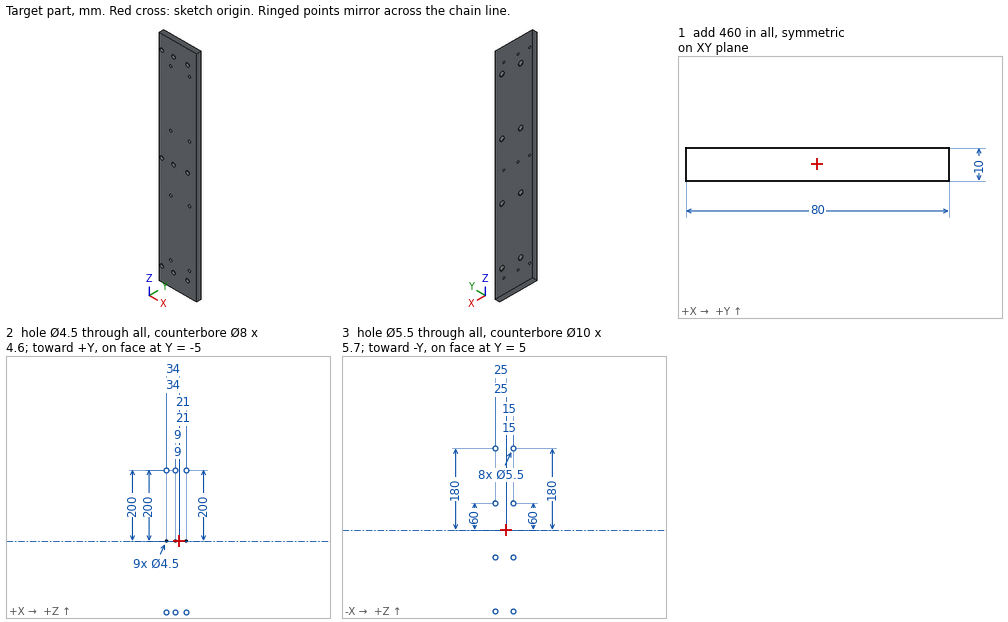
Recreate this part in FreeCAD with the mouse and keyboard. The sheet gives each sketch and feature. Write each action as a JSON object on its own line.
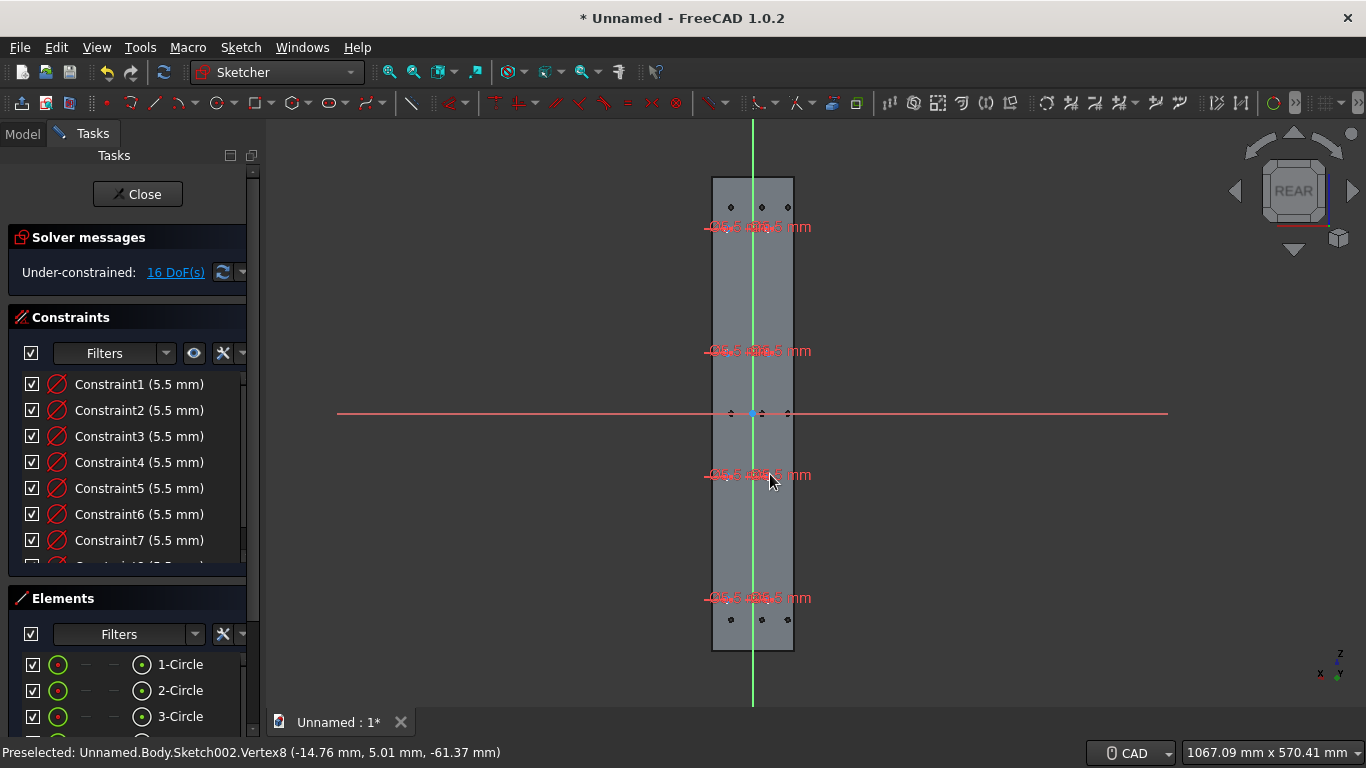
{"action": "left_click", "coordinate": [727, 353]}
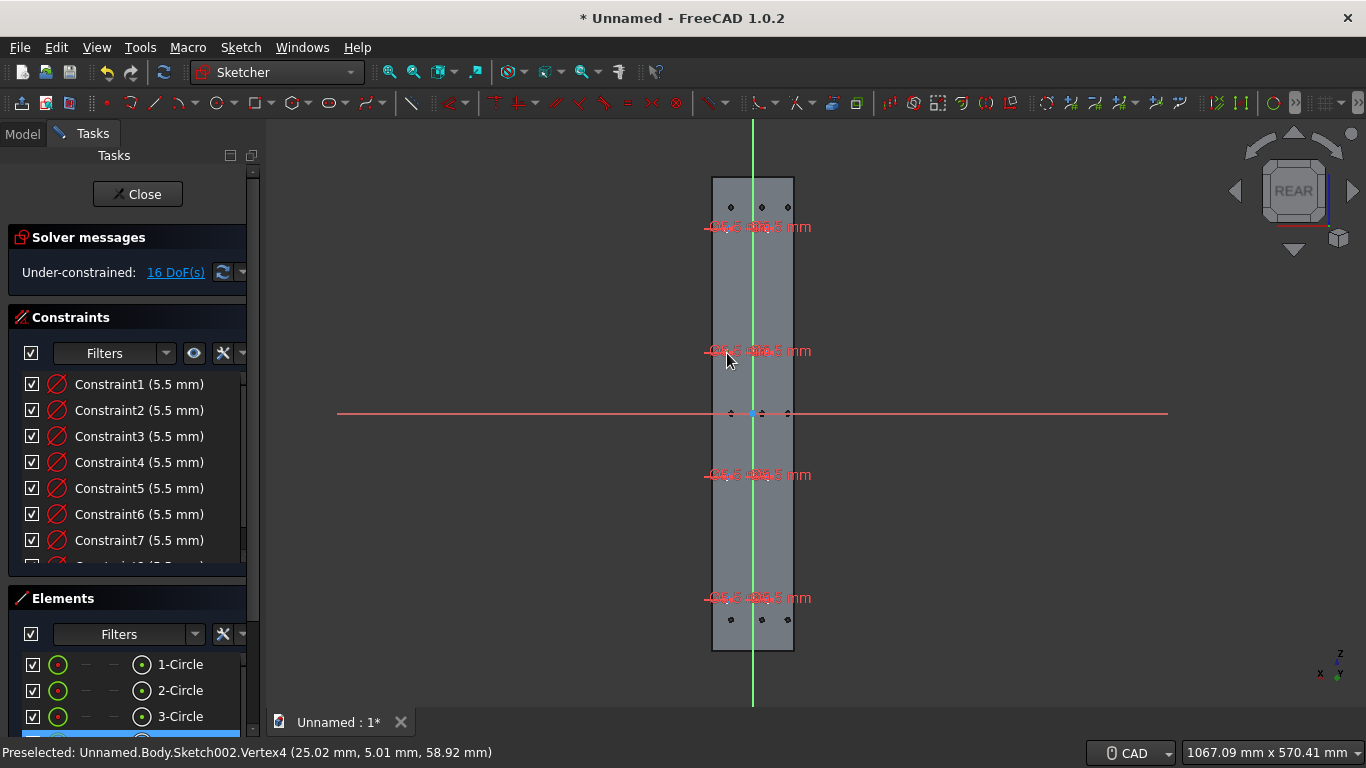
{"action": "left_click", "coordinate": [727, 477]}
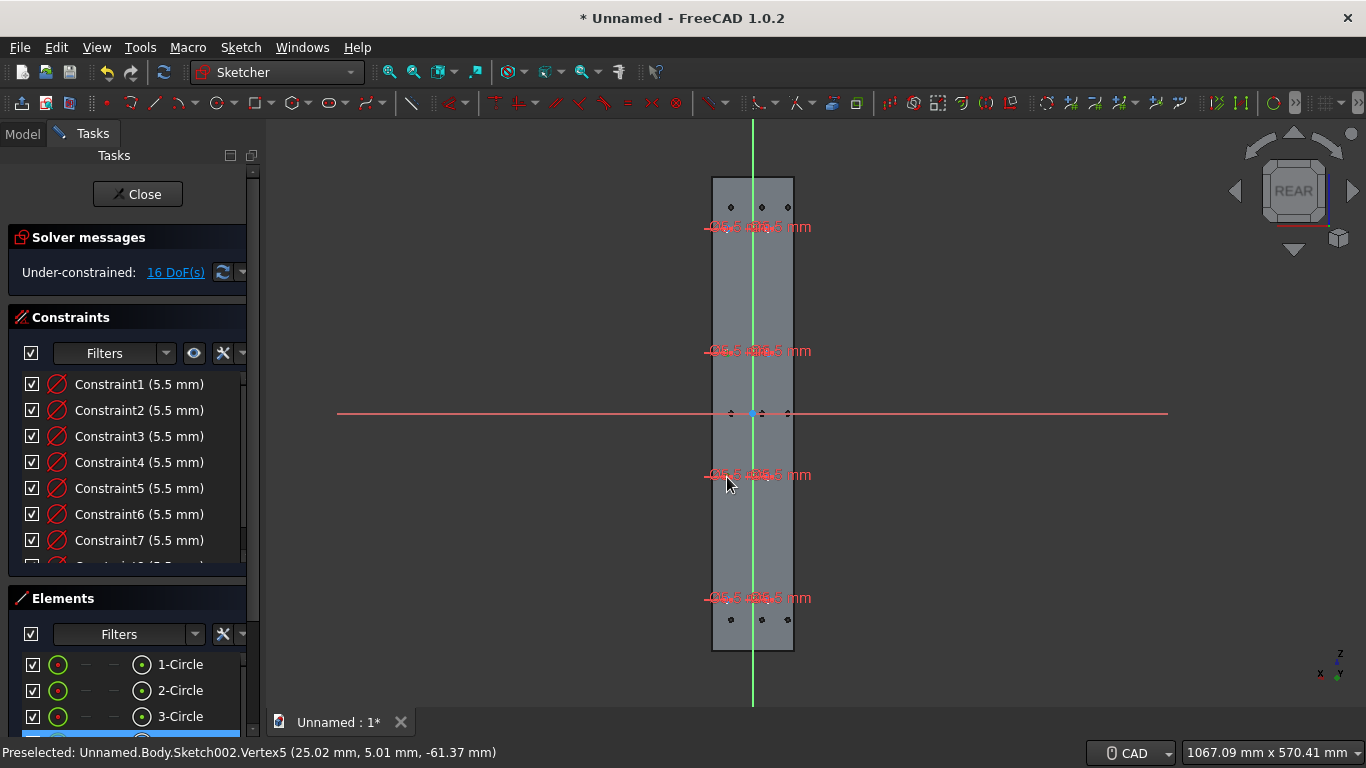
{"action": "left_click", "coordinate": [359, 414]}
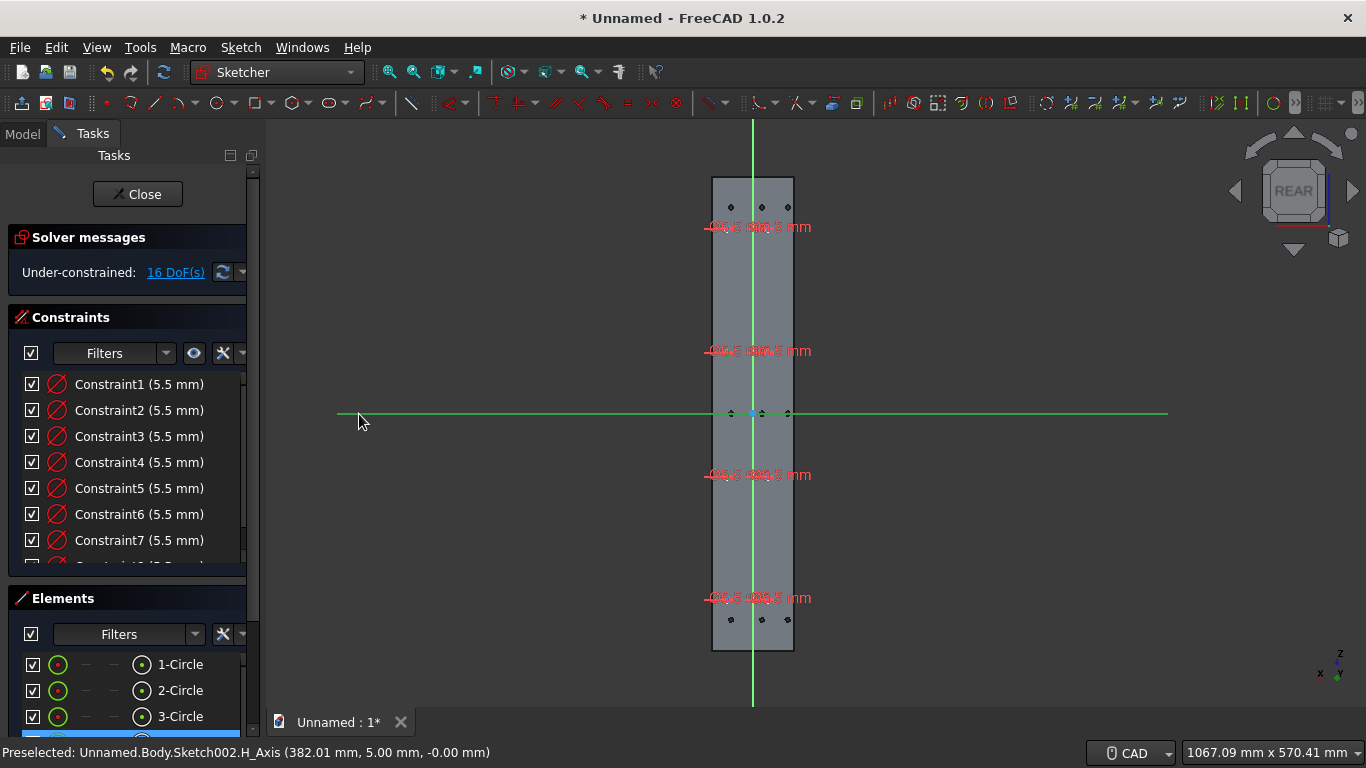
{"action": "key", "text": "s"}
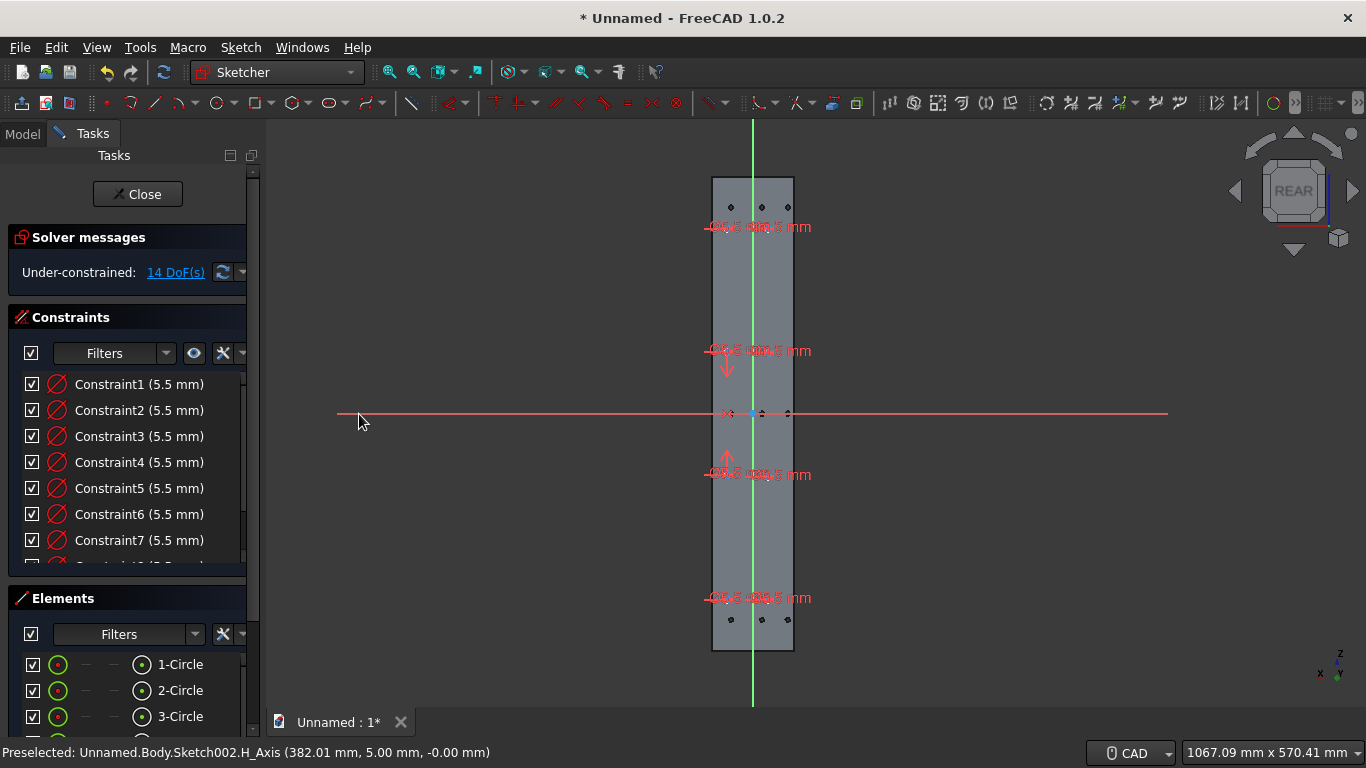
{"action": "left_click", "coordinate": [727, 229]}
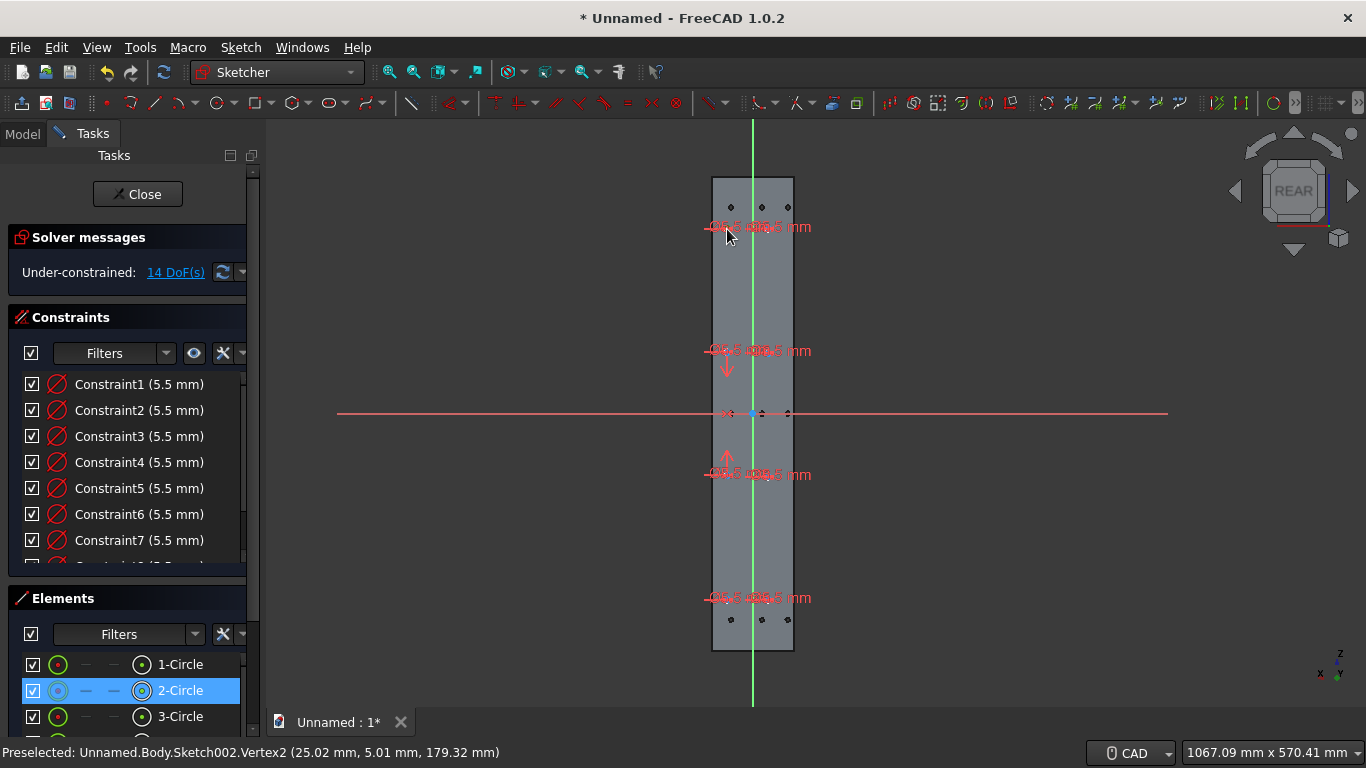
{"action": "left_click", "coordinate": [727, 600]}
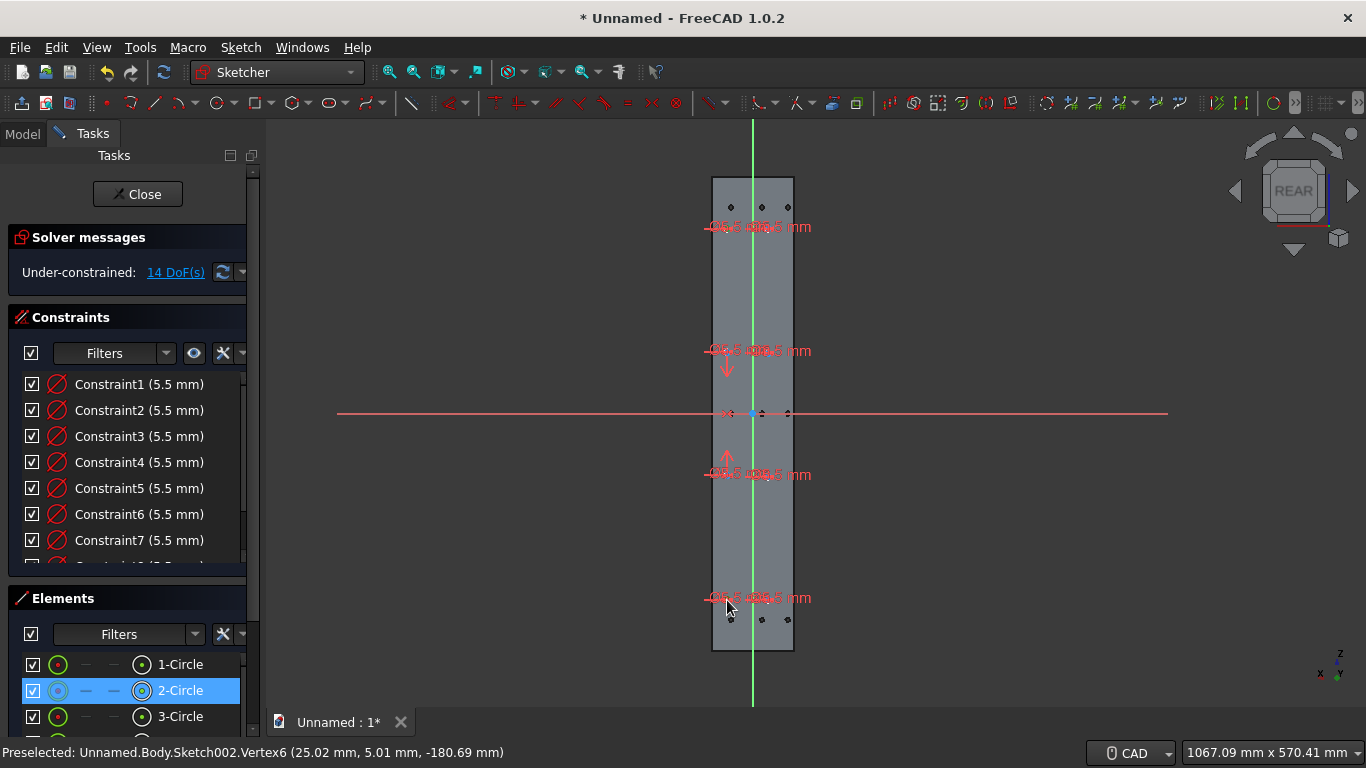
{"action": "left_click", "coordinate": [359, 414]}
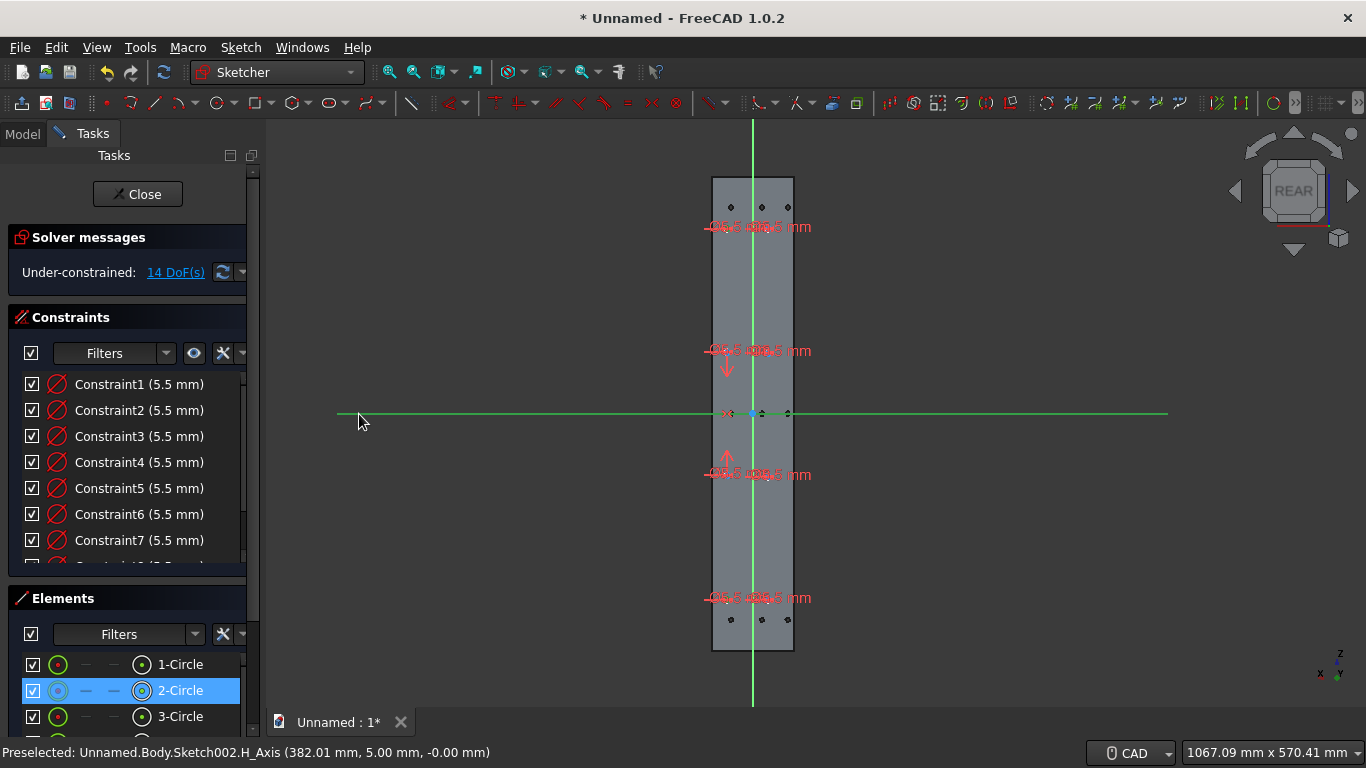
{"action": "left_click", "coordinate": [652, 104]}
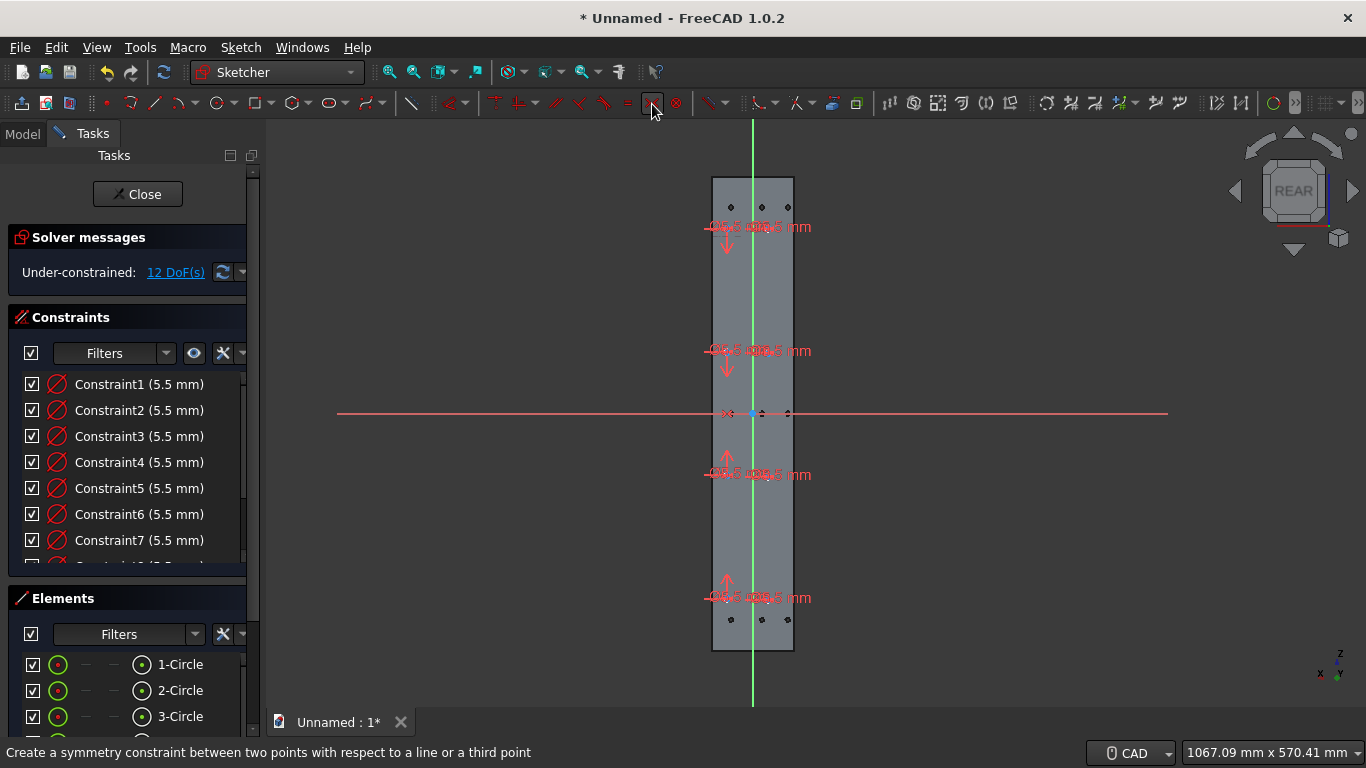
{"action": "left_click", "coordinate": [768, 229]}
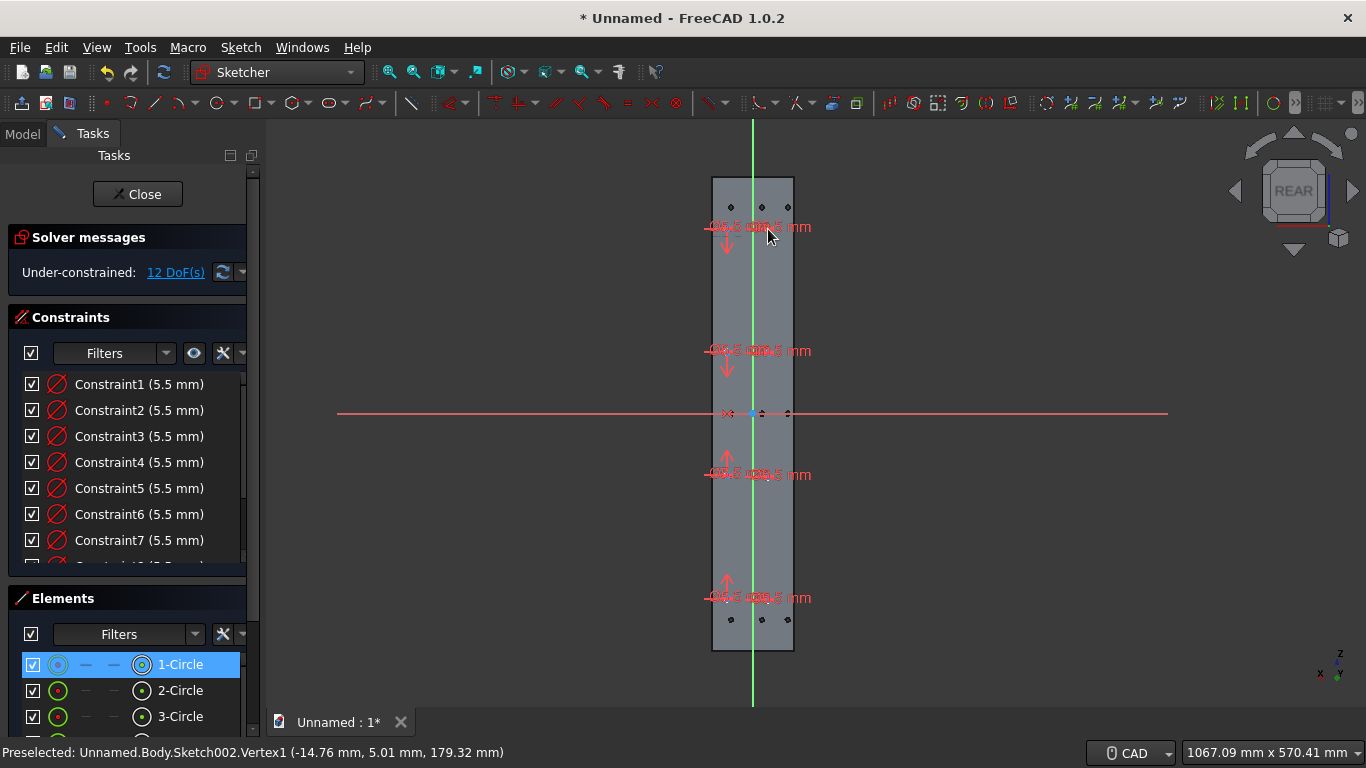
{"action": "left_click", "coordinate": [768, 600]}